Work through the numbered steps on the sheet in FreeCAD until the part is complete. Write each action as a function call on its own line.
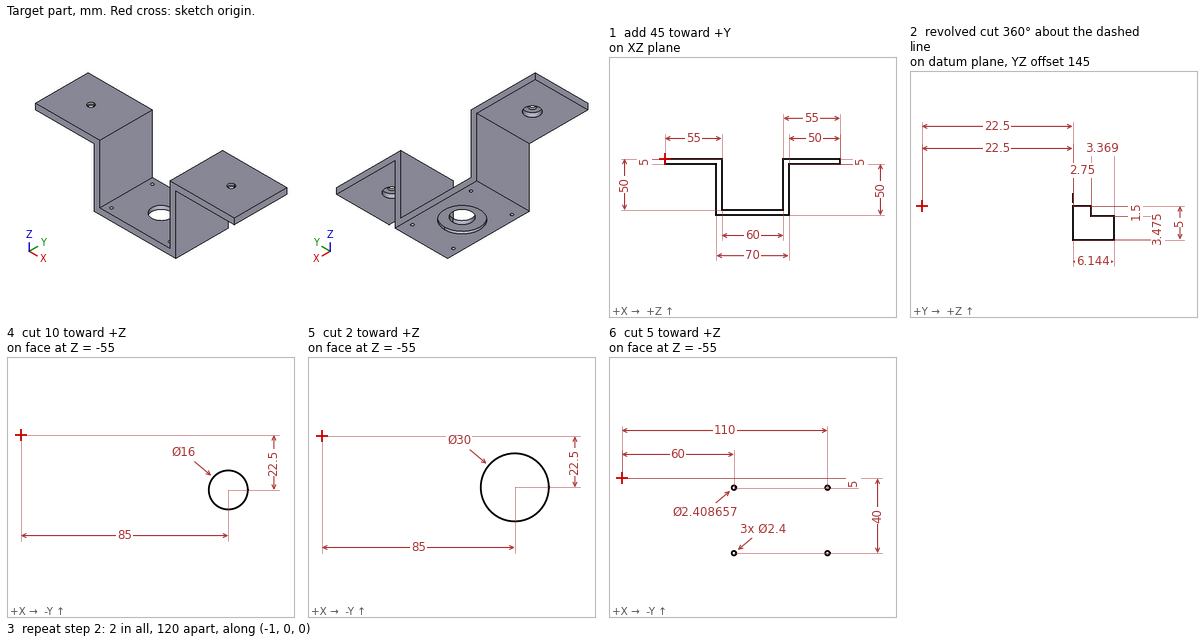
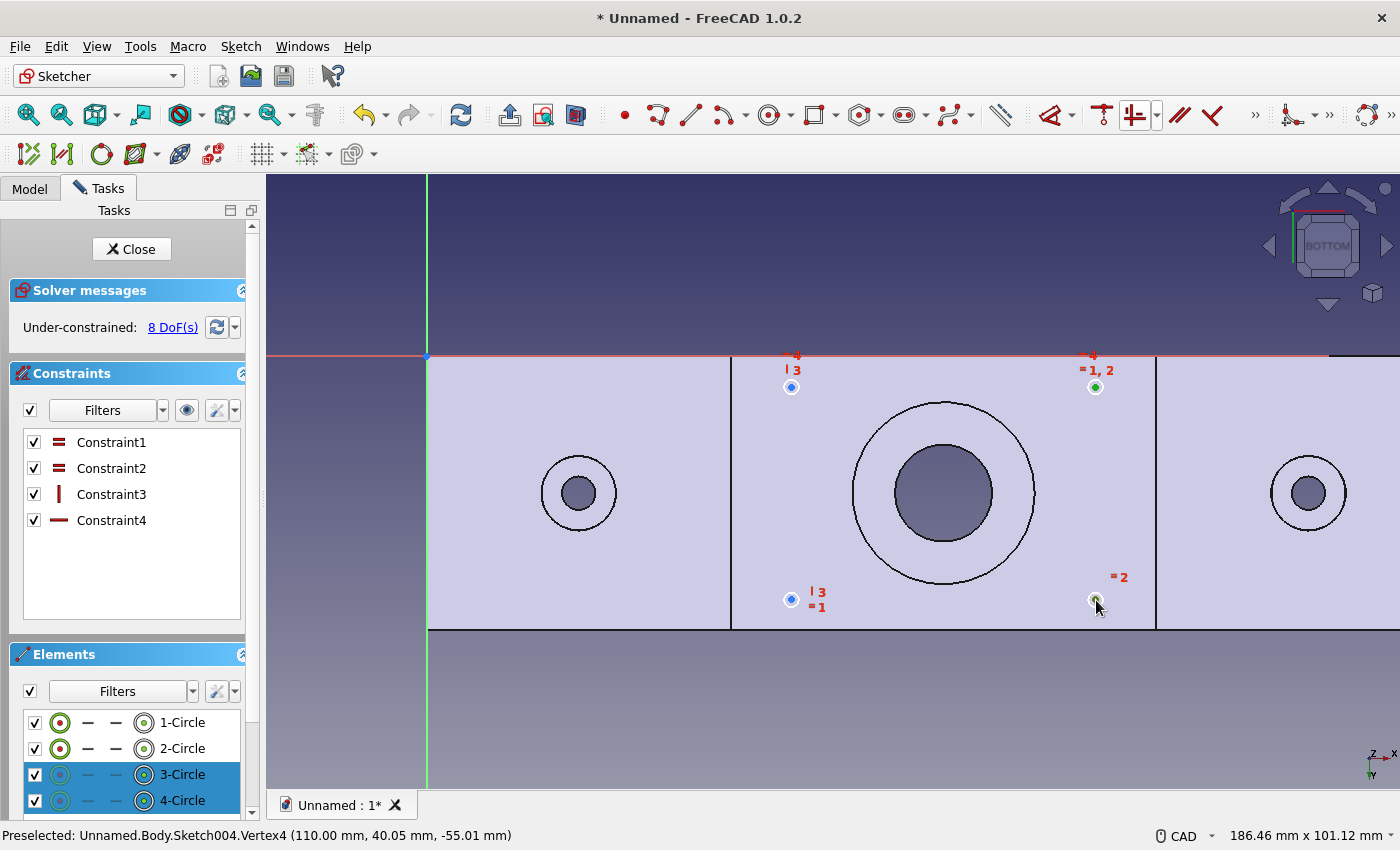
click(1156, 116)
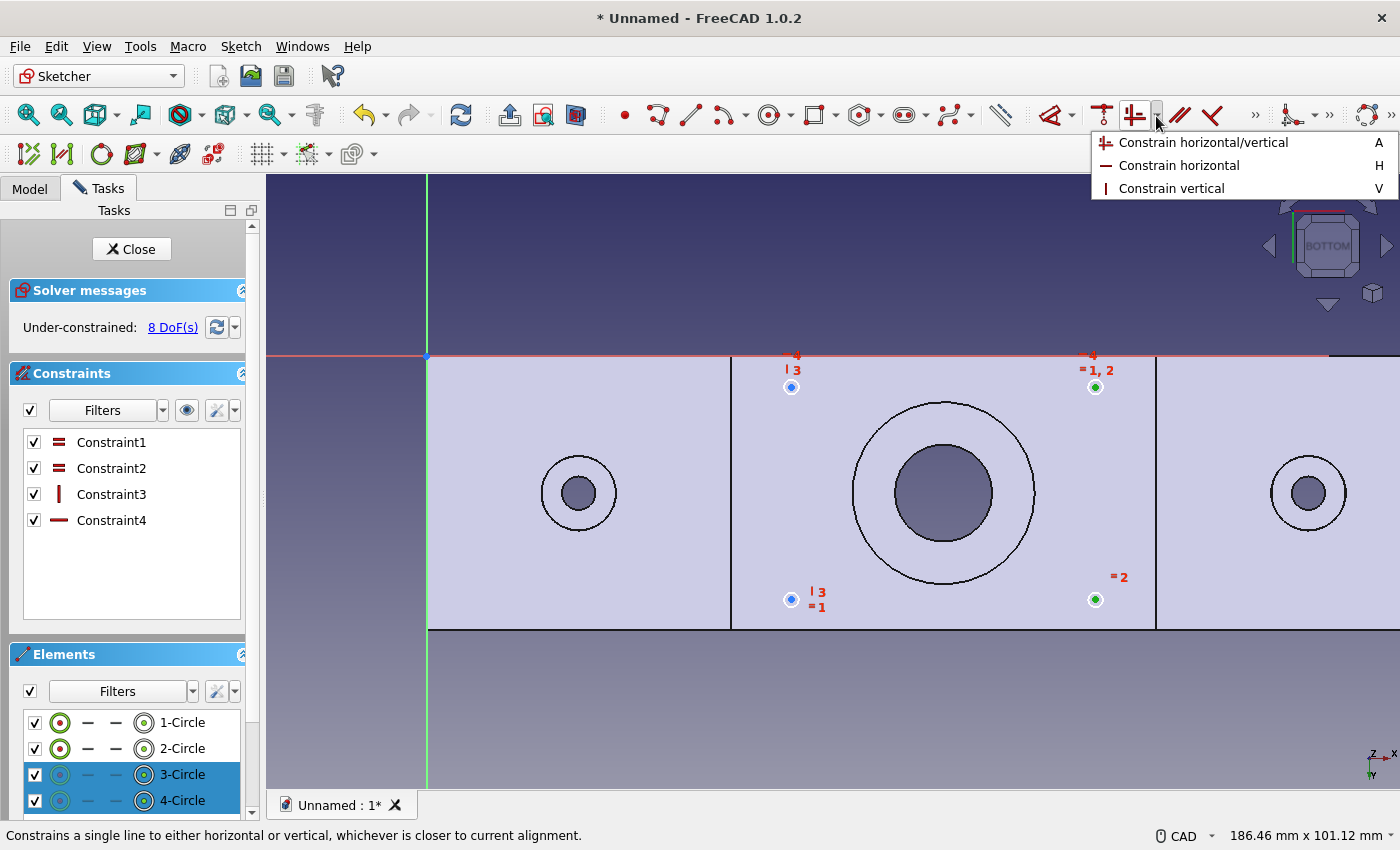
click(1245, 188)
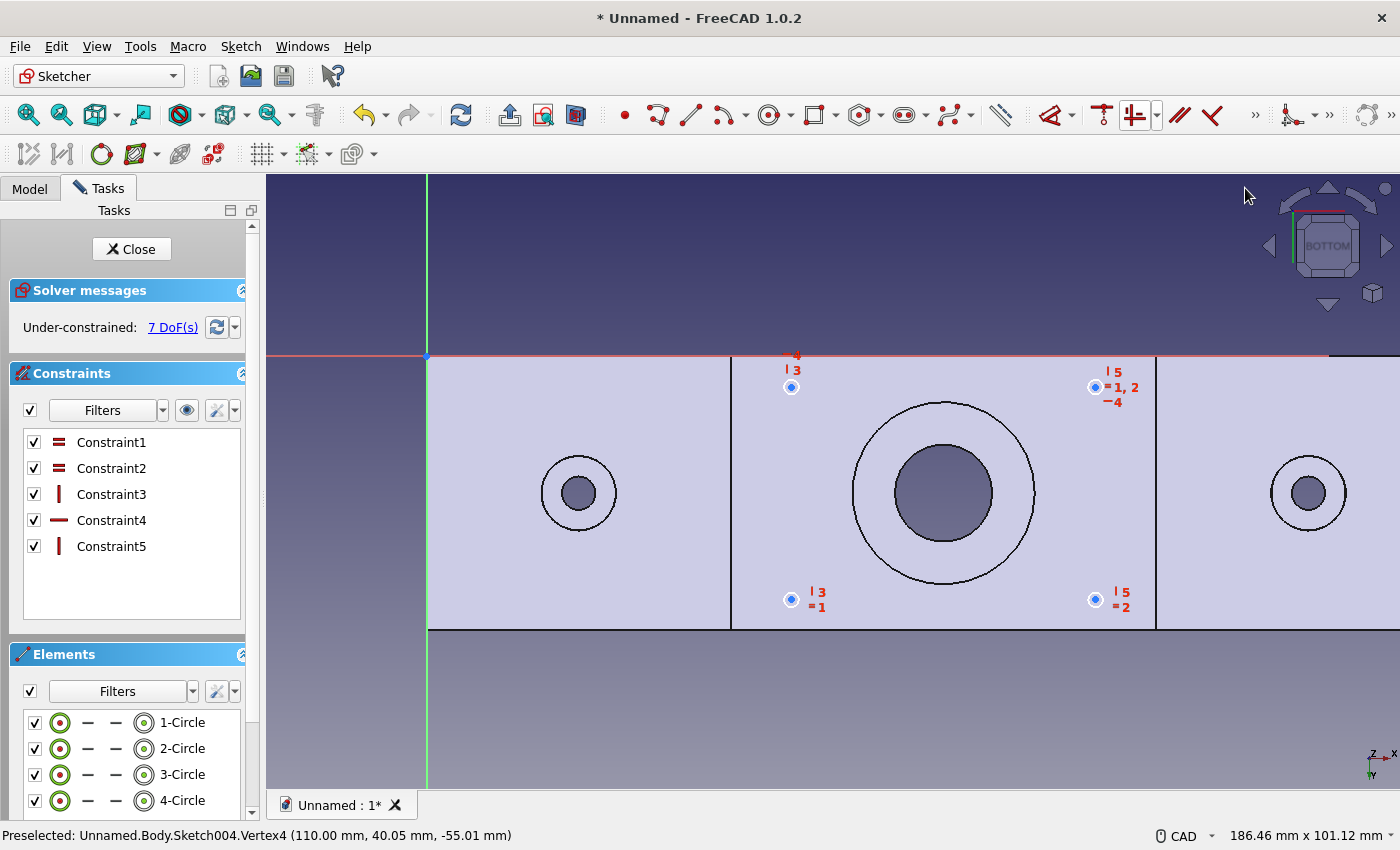
click(791, 600)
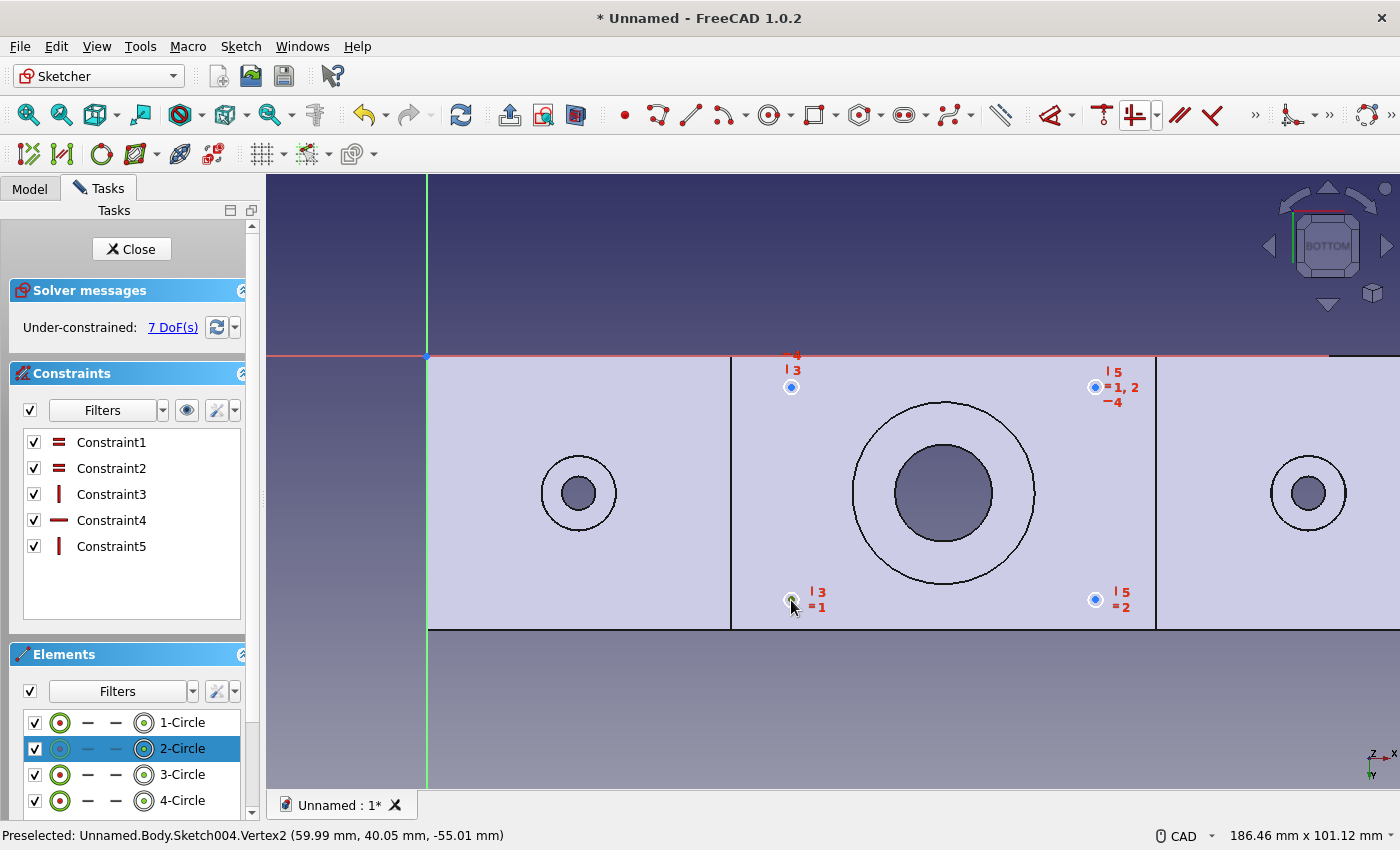
click(1096, 600)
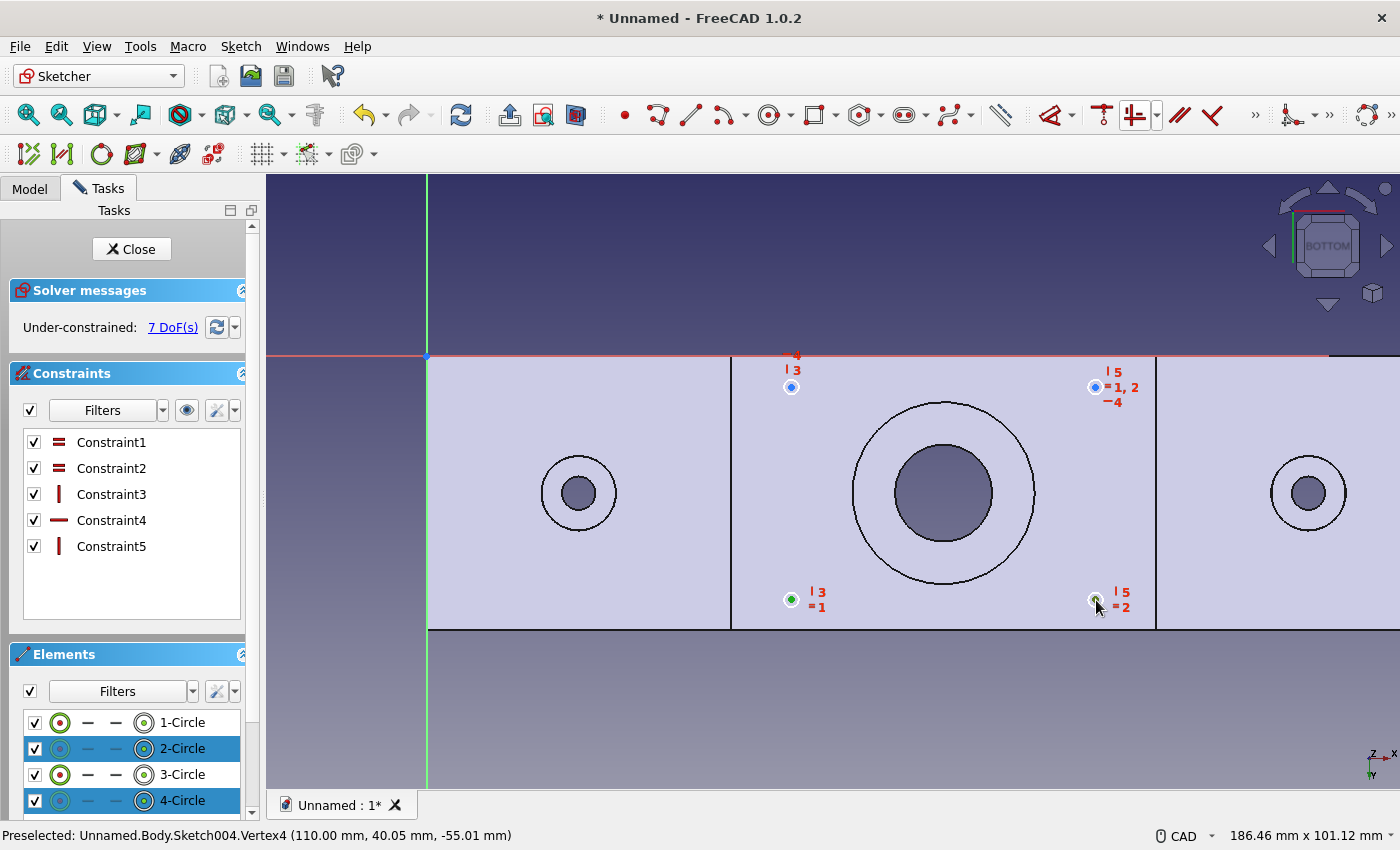
key(h)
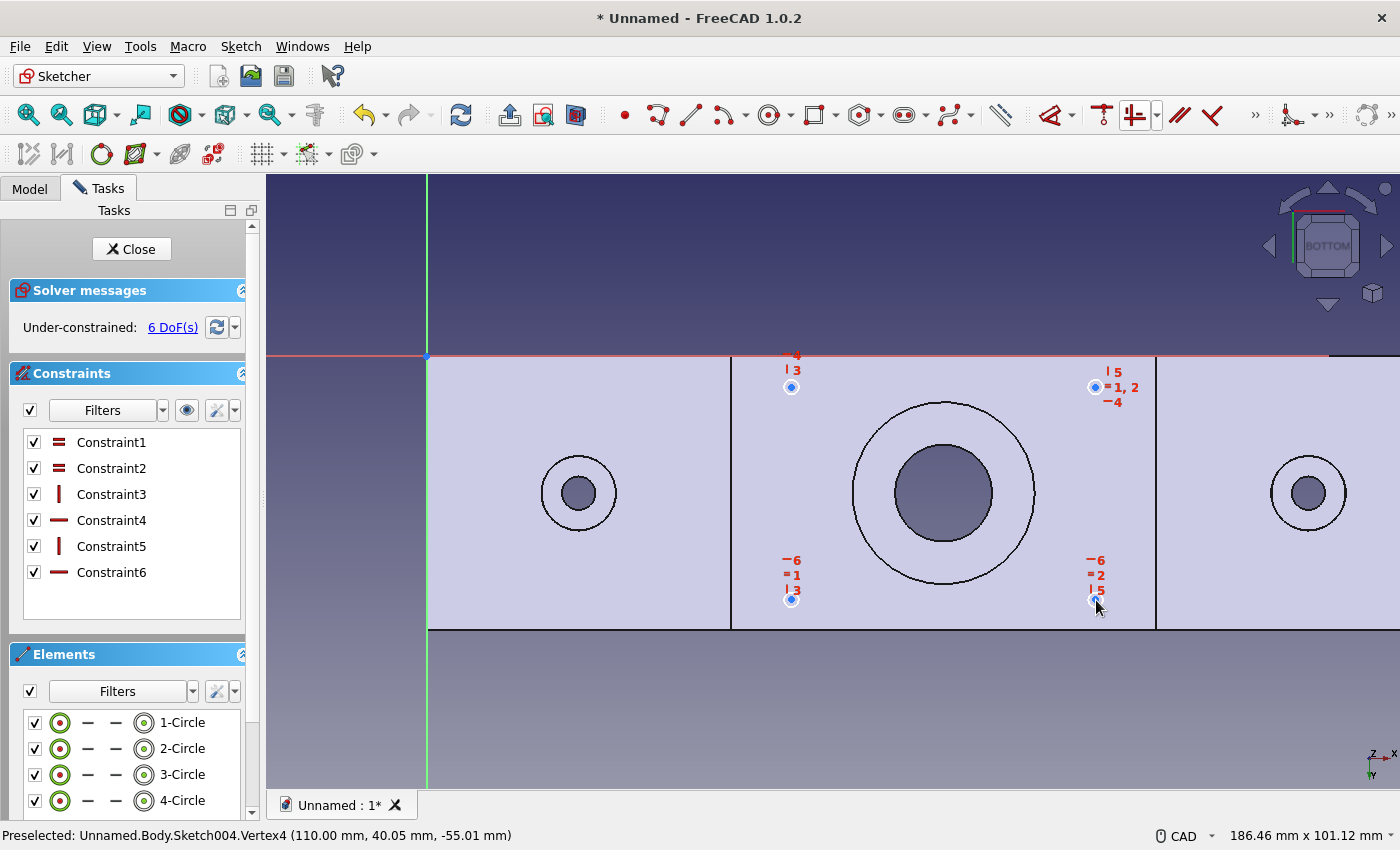
key(d)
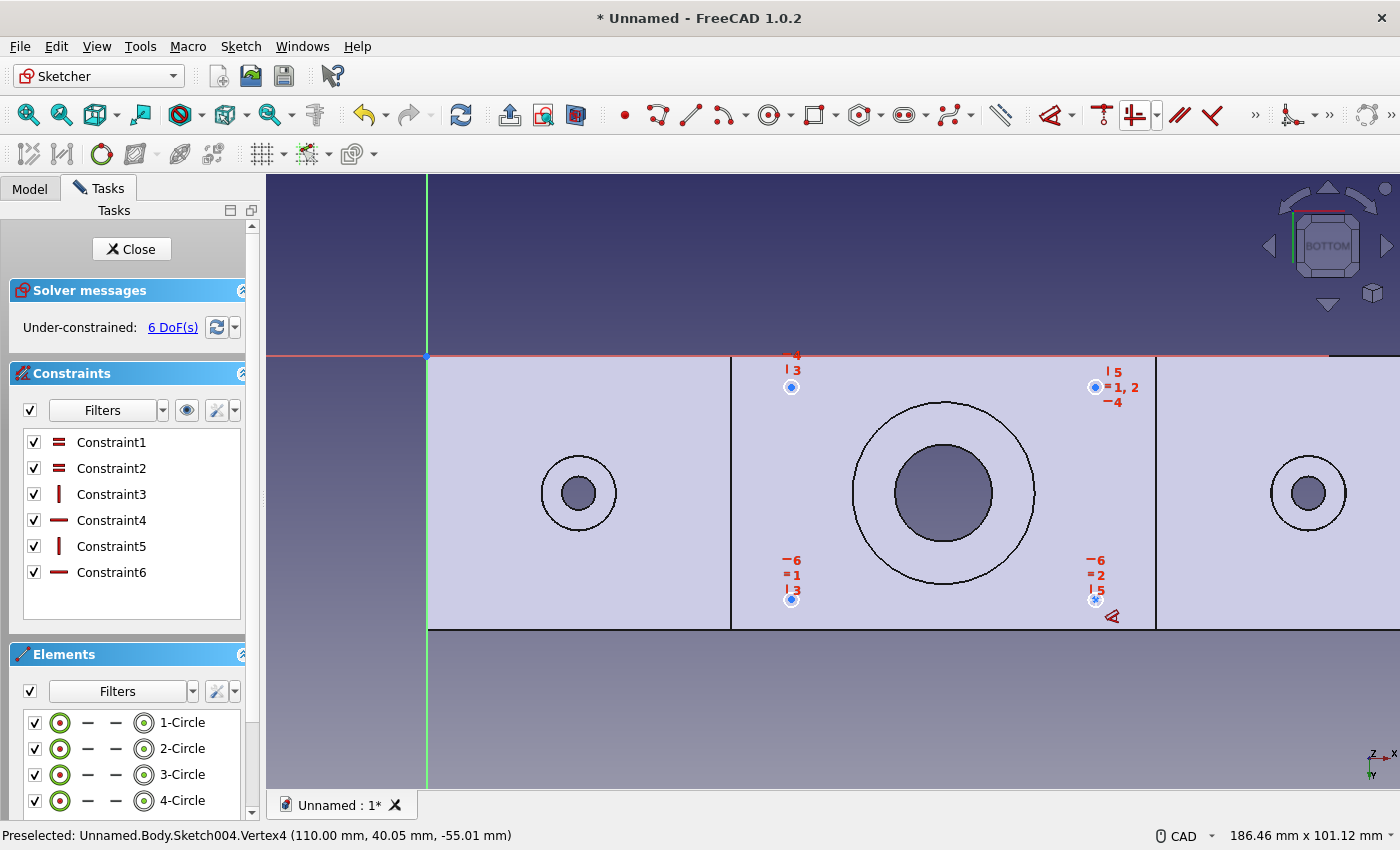
scroll(797, 382, up, 5)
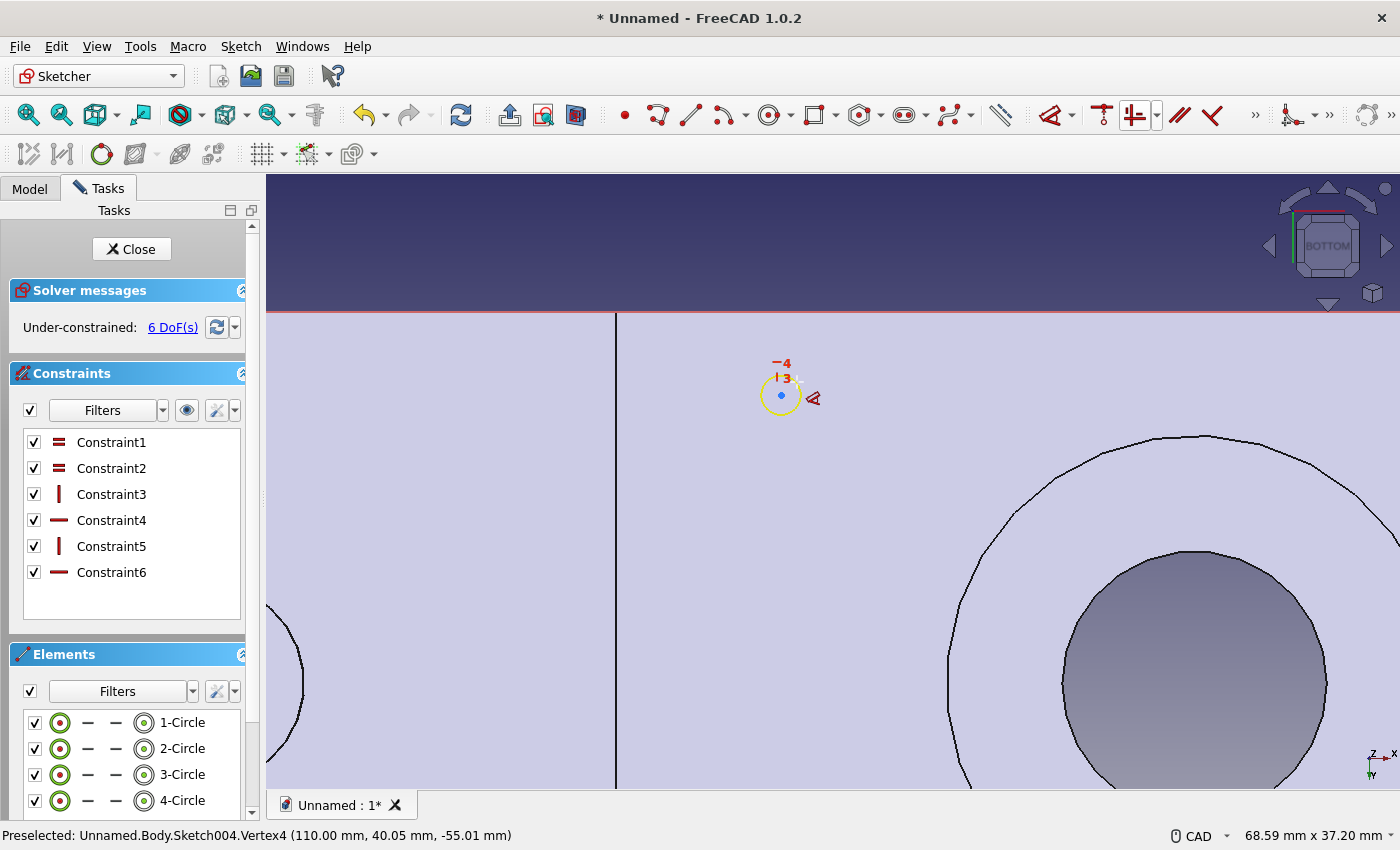
click(795, 381)
click(817, 358)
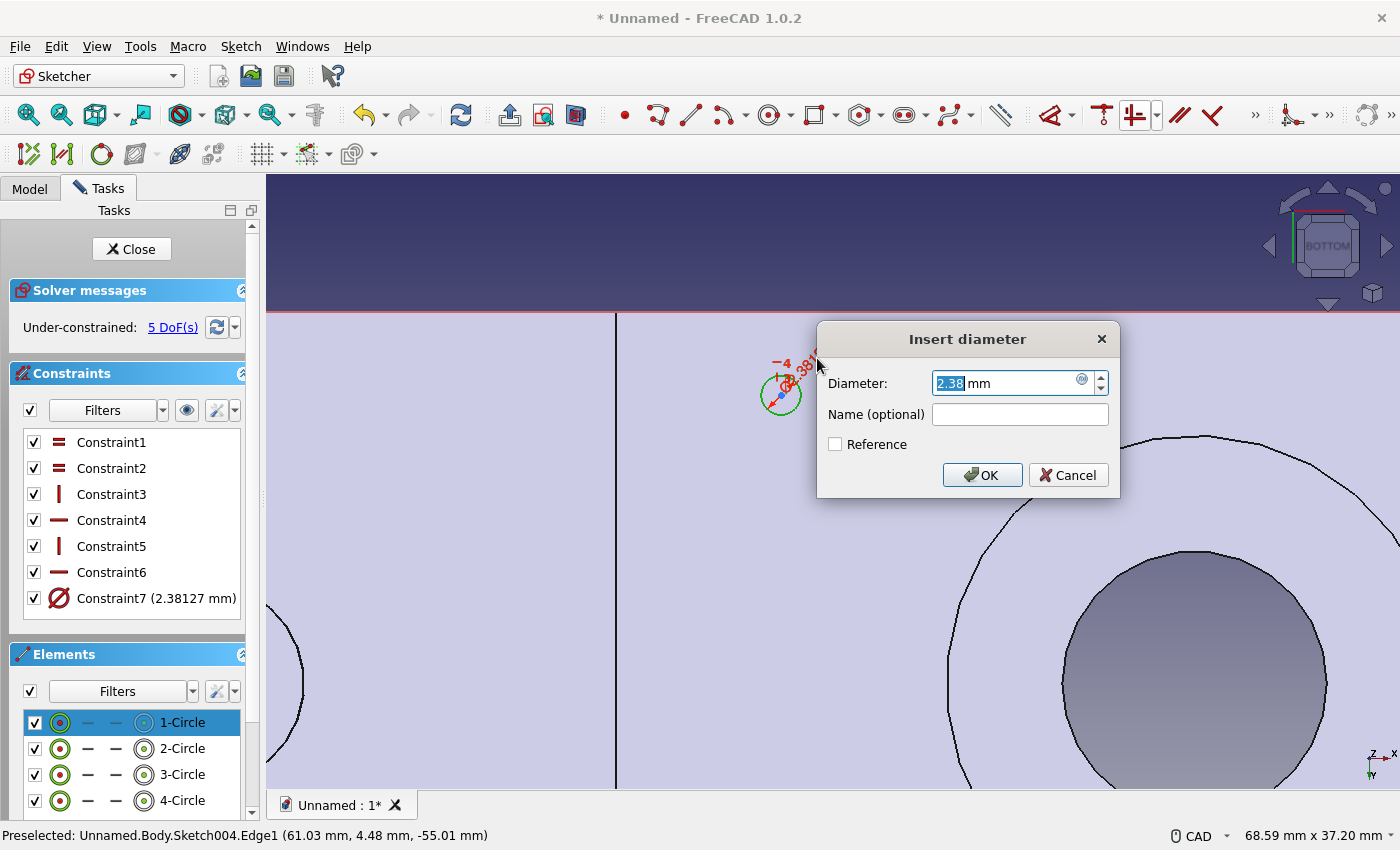
text(2.408657)
key(Return)